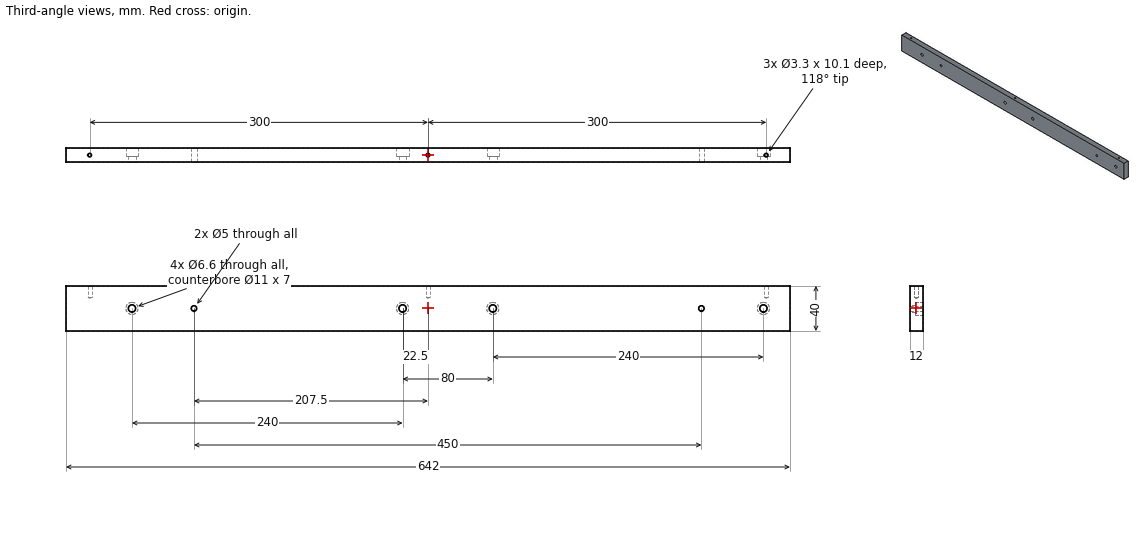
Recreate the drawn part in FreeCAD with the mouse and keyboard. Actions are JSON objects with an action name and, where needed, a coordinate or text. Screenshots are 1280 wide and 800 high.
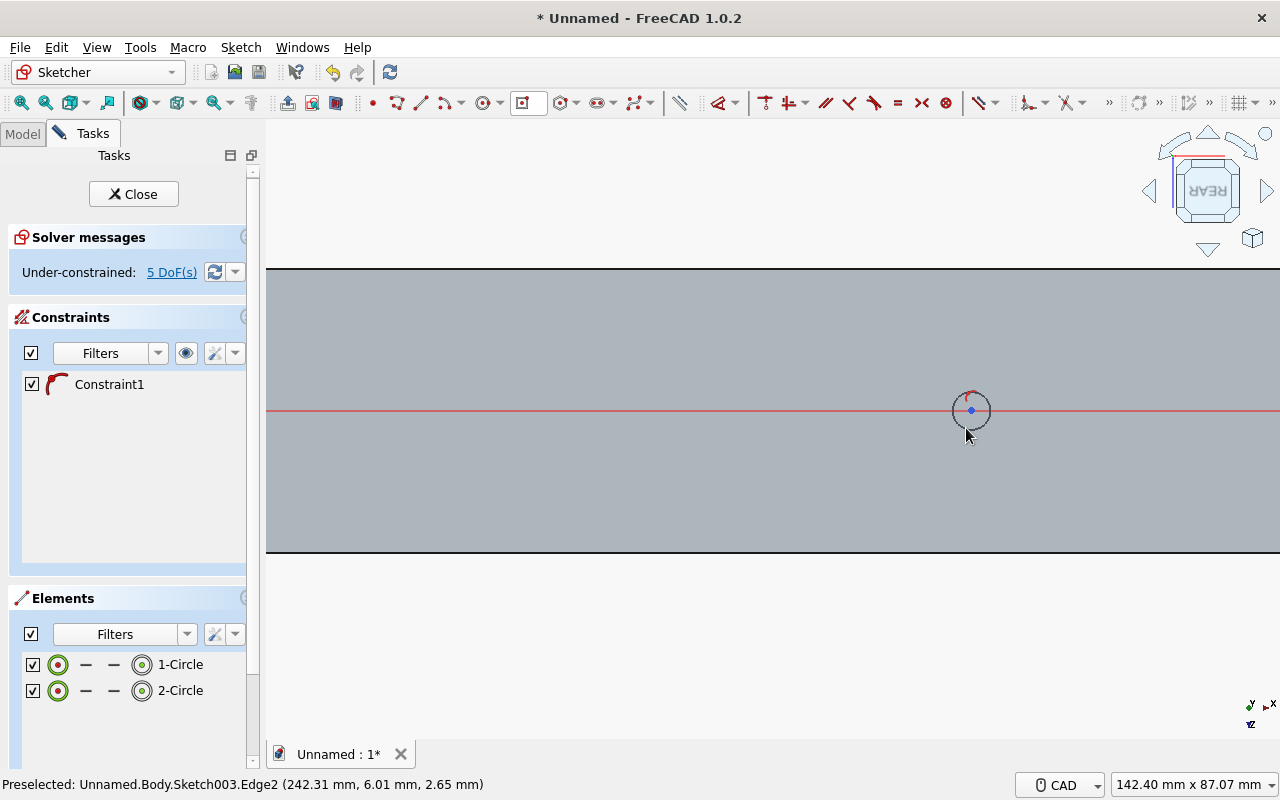
{"action": "scroll", "coordinate": [969, 433], "scroll_direction": "down", "scroll_amount": 9}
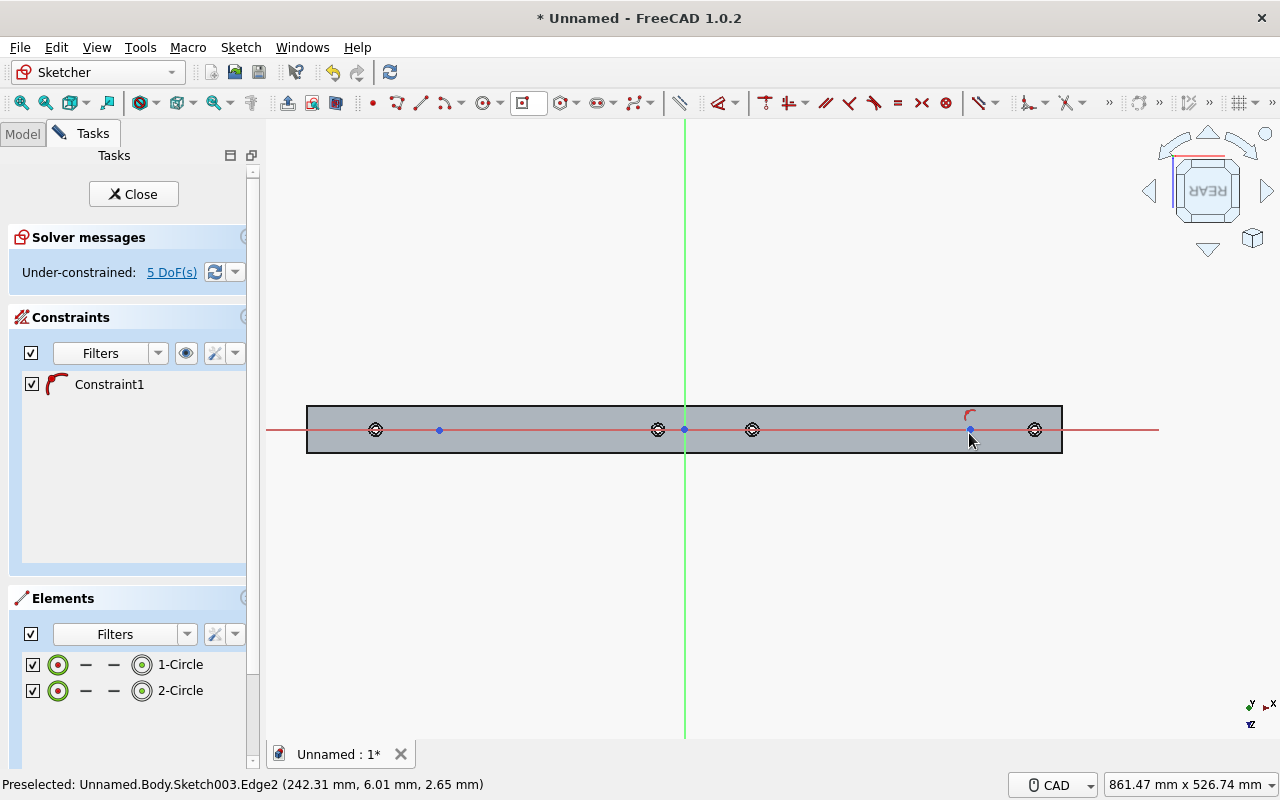
{"action": "scroll", "coordinate": [441, 430], "scroll_direction": "up", "scroll_amount": 11}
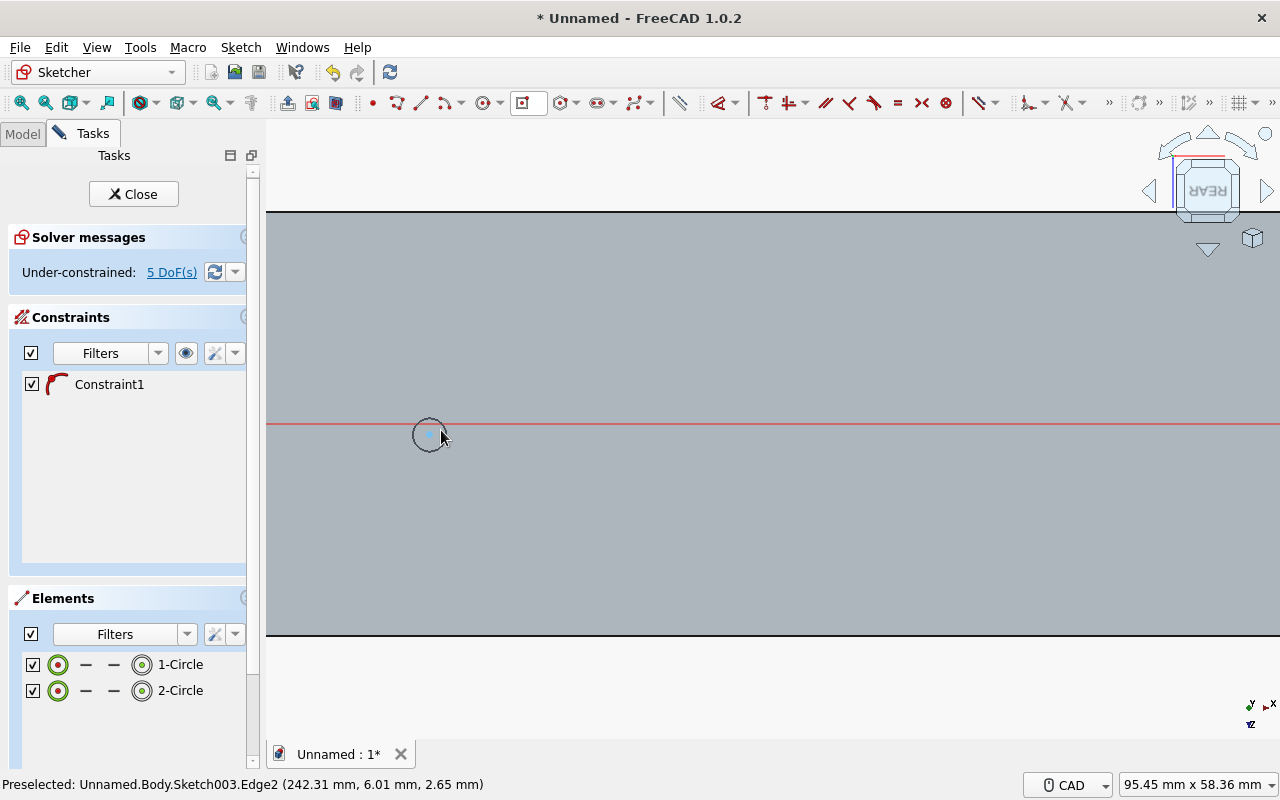
{"action": "left_click", "coordinate": [441, 423]}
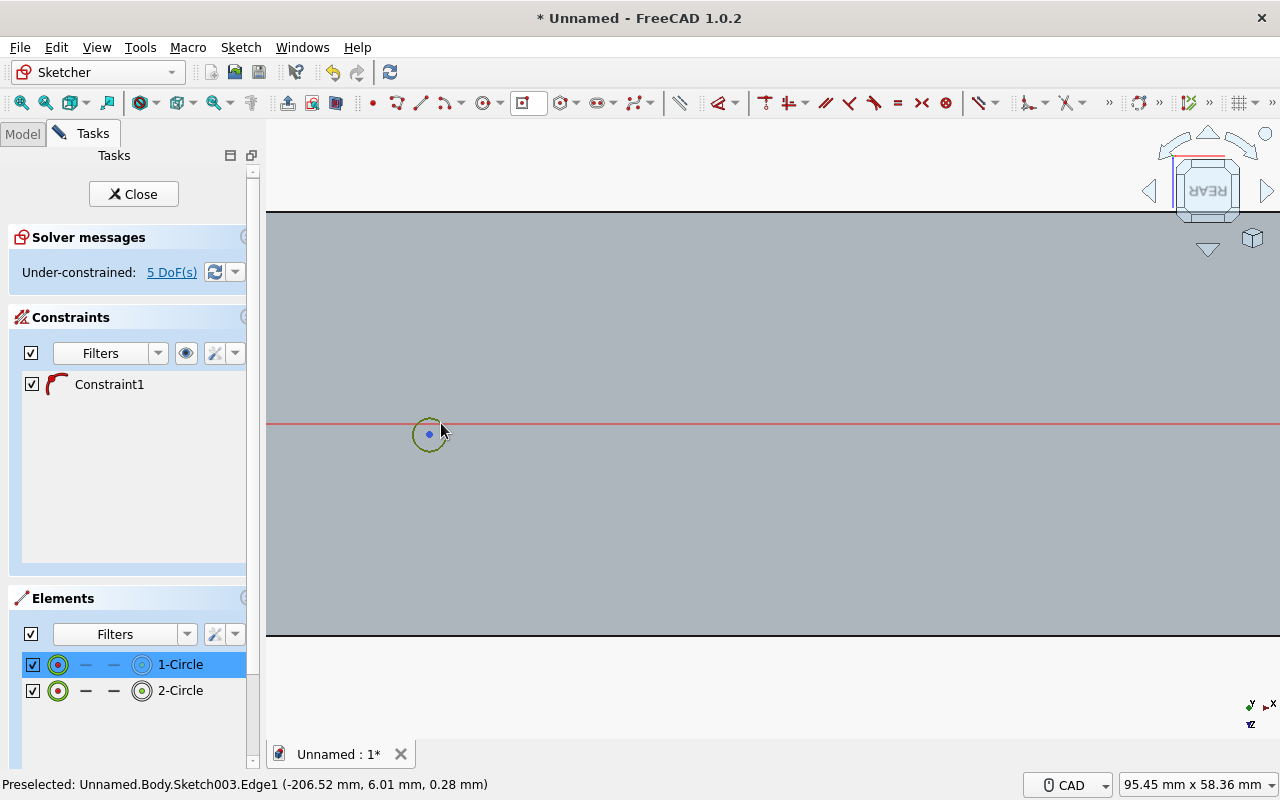
{"action": "scroll", "coordinate": [440, 430], "scroll_direction": "down", "scroll_amount": 11}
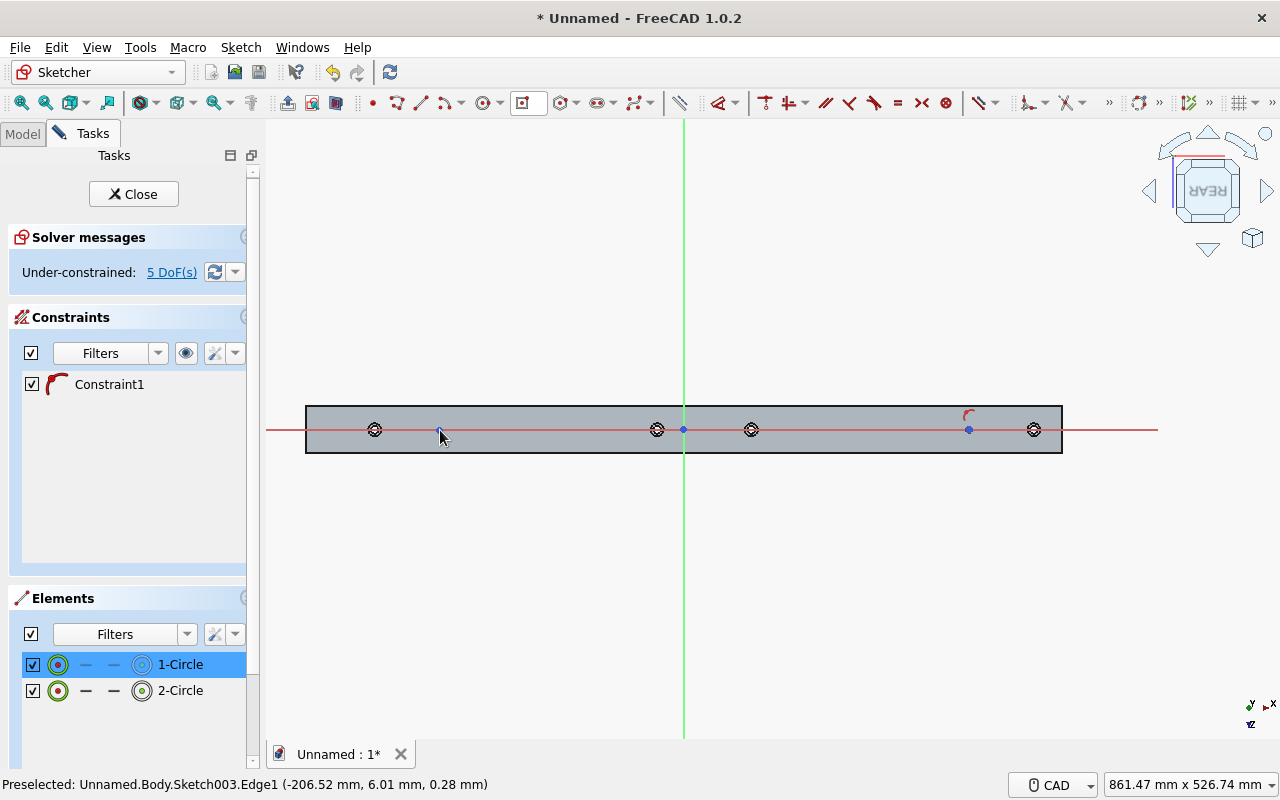
{"action": "scroll", "coordinate": [971, 428], "scroll_direction": "up", "scroll_amount": 10}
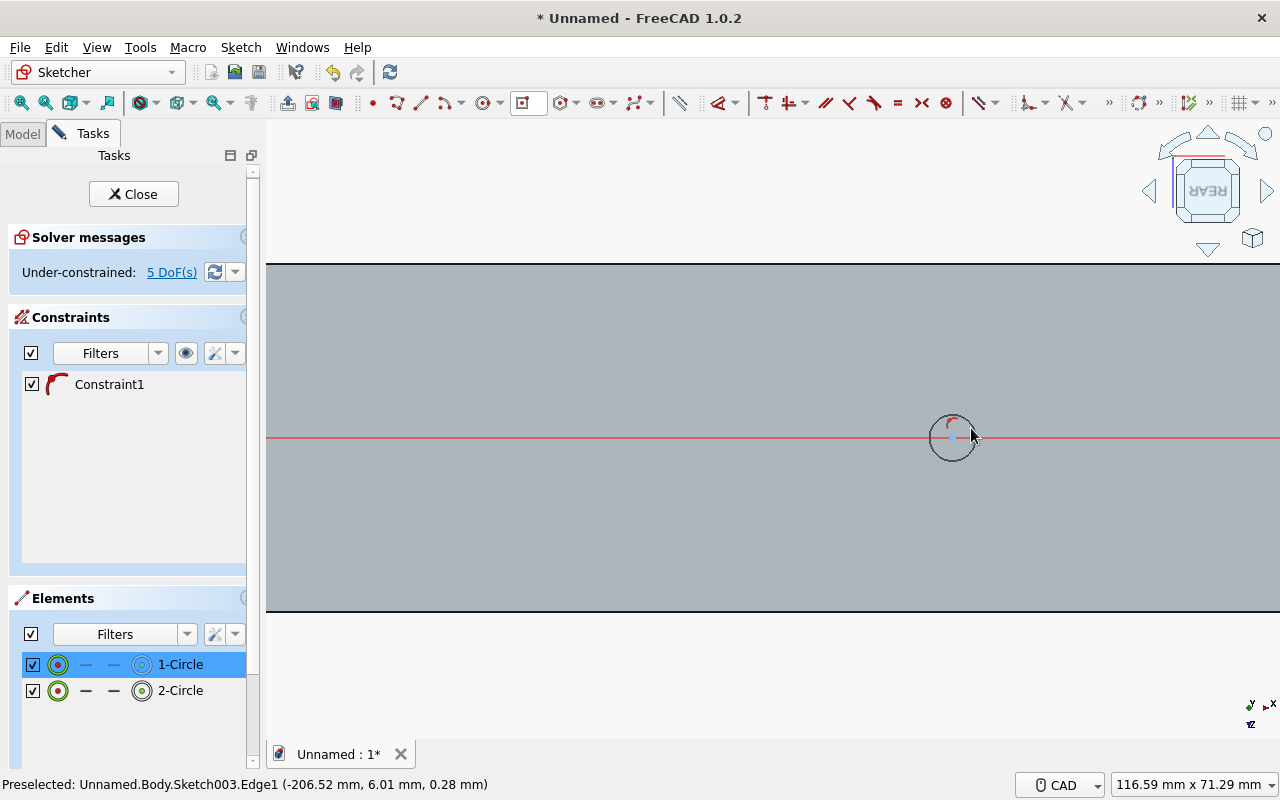
{"action": "left_click", "coordinate": [969, 422]}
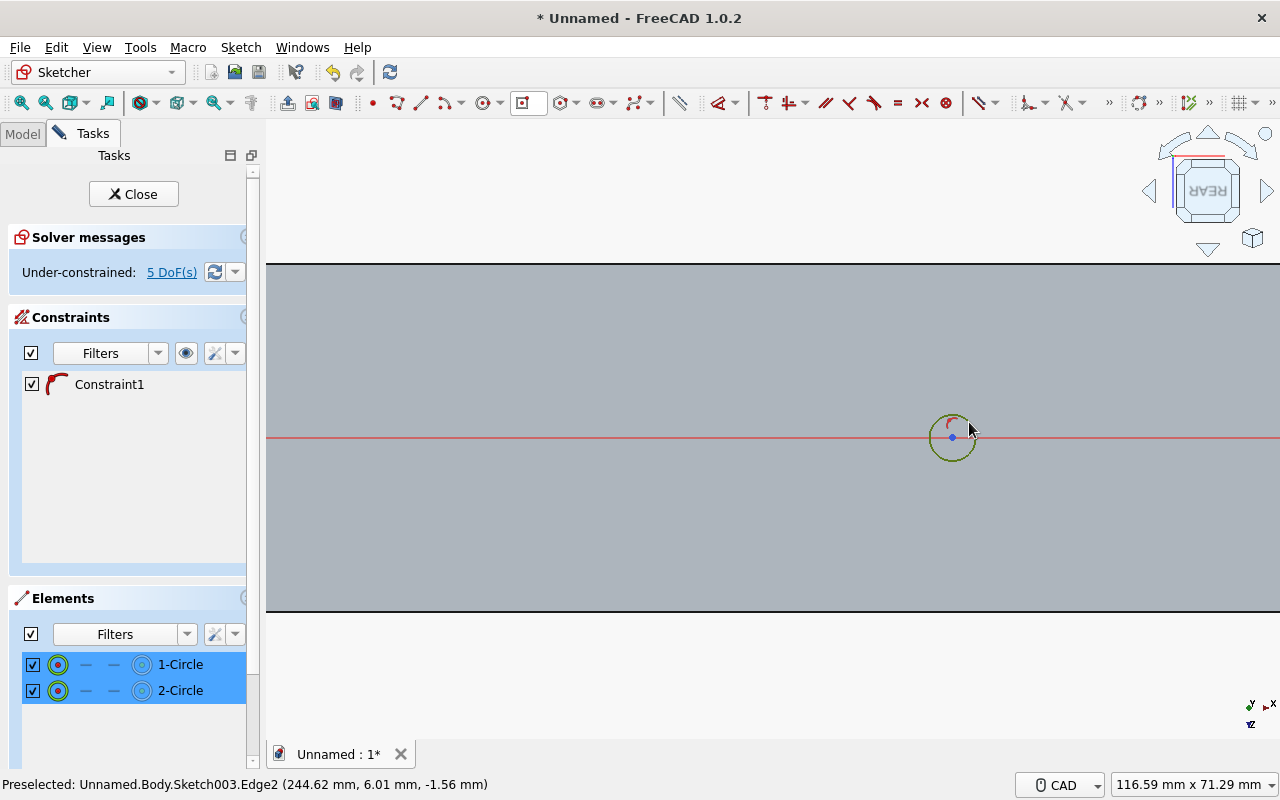
{"action": "left_click", "coordinate": [898, 104]}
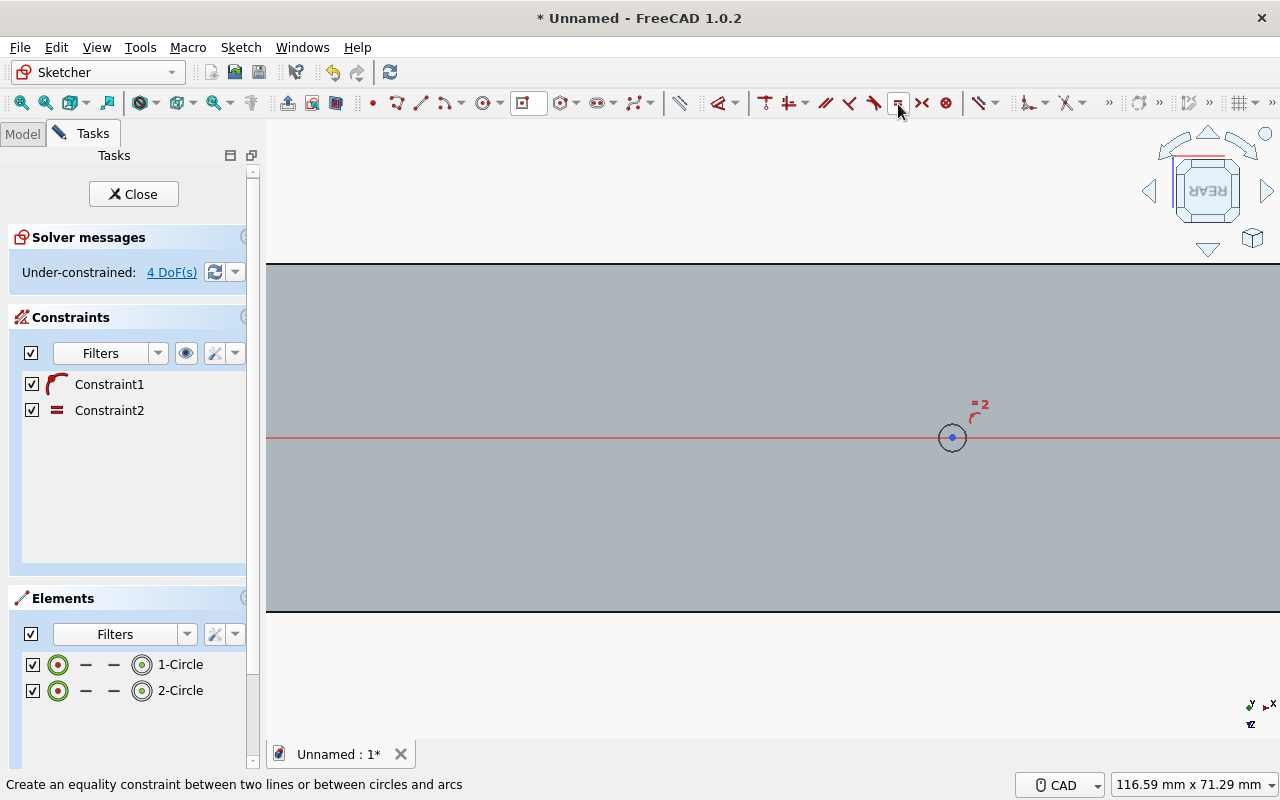
{"action": "scroll", "coordinate": [972, 428], "scroll_direction": "down", "scroll_amount": 10}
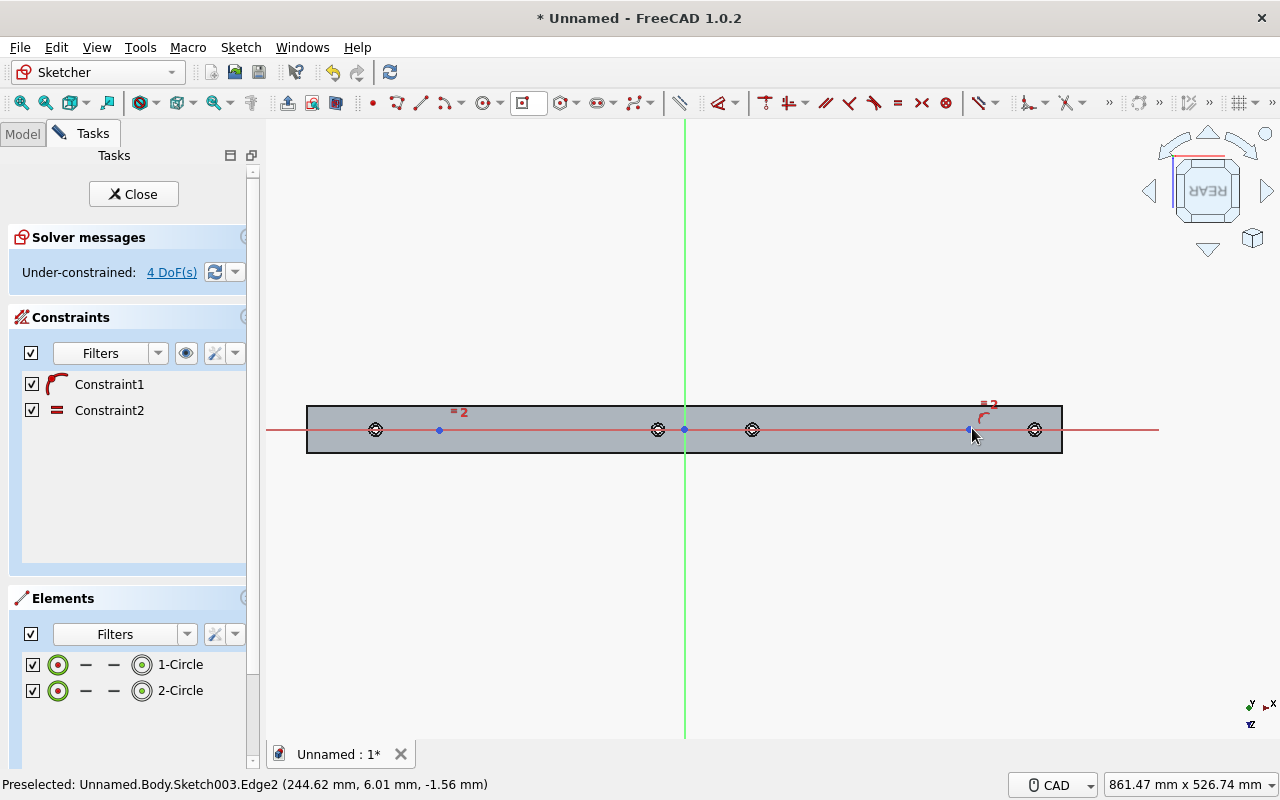
{"action": "left_click", "coordinate": [440, 431]}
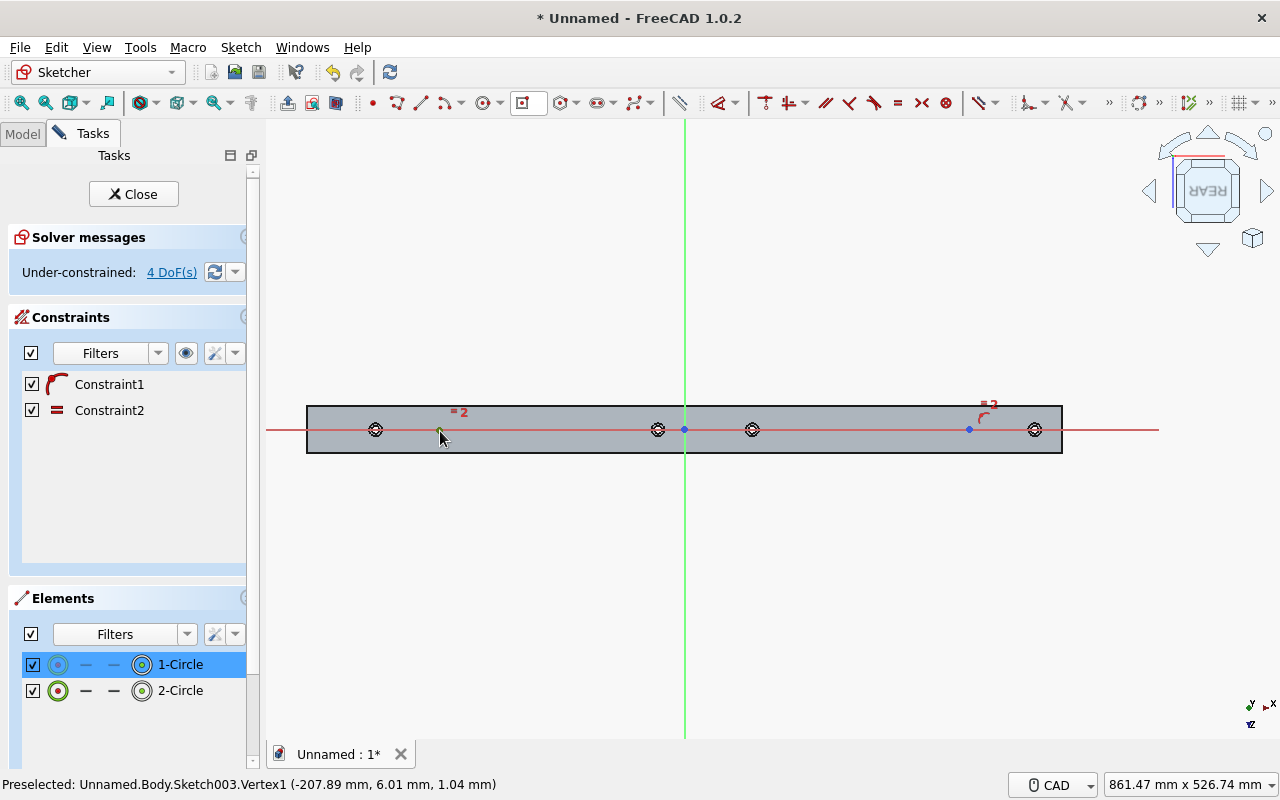
{"action": "left_click", "coordinate": [353, 430]}